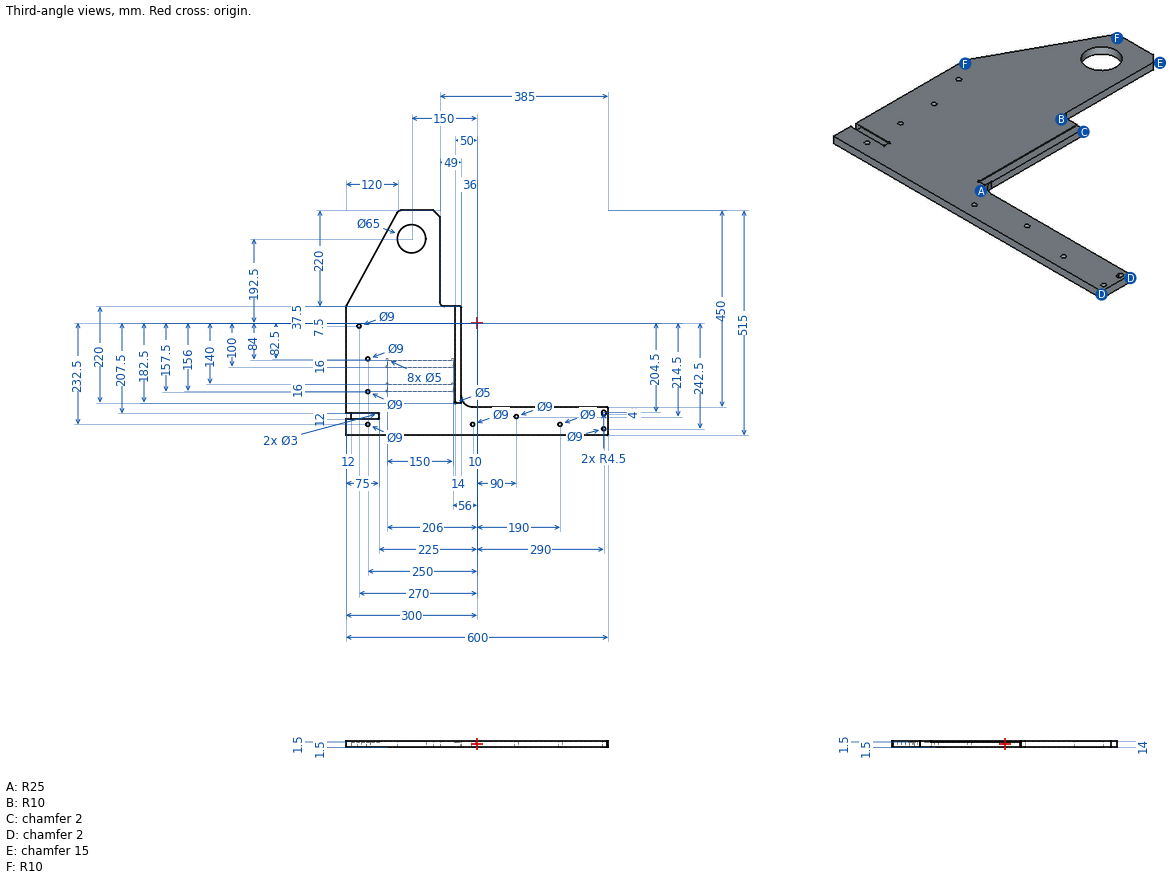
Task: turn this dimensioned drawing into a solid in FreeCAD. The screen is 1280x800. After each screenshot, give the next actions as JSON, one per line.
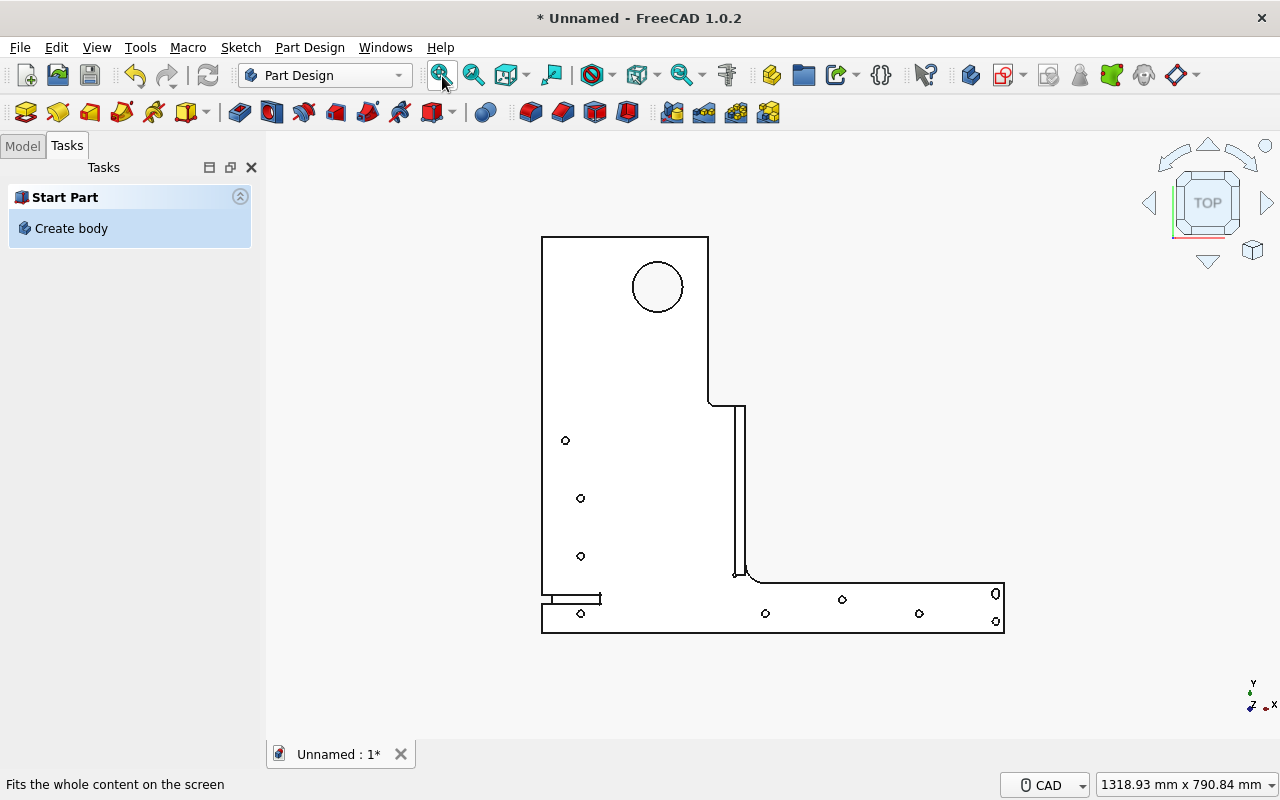
{"action": "key", "text": "0"}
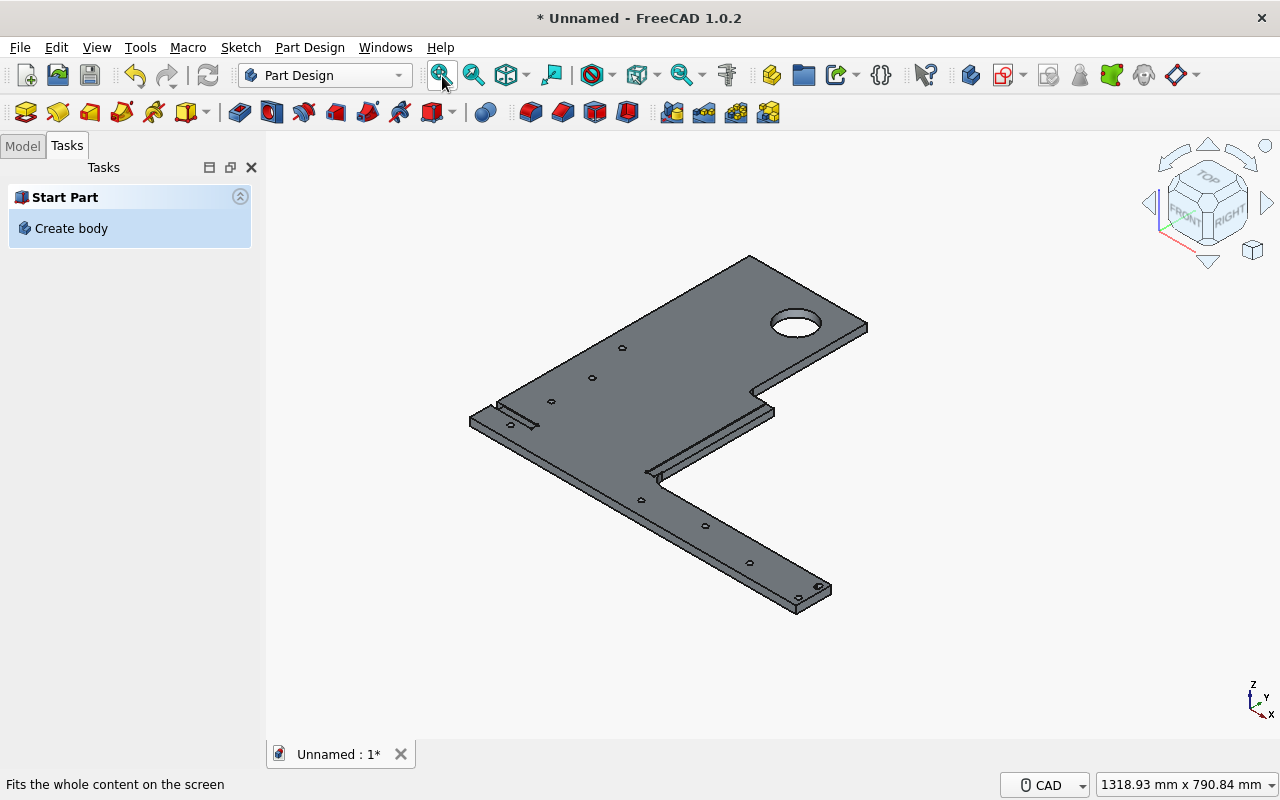
{"action": "scroll", "coordinate": [774, 411], "scroll_direction": "up", "scroll_amount": 8}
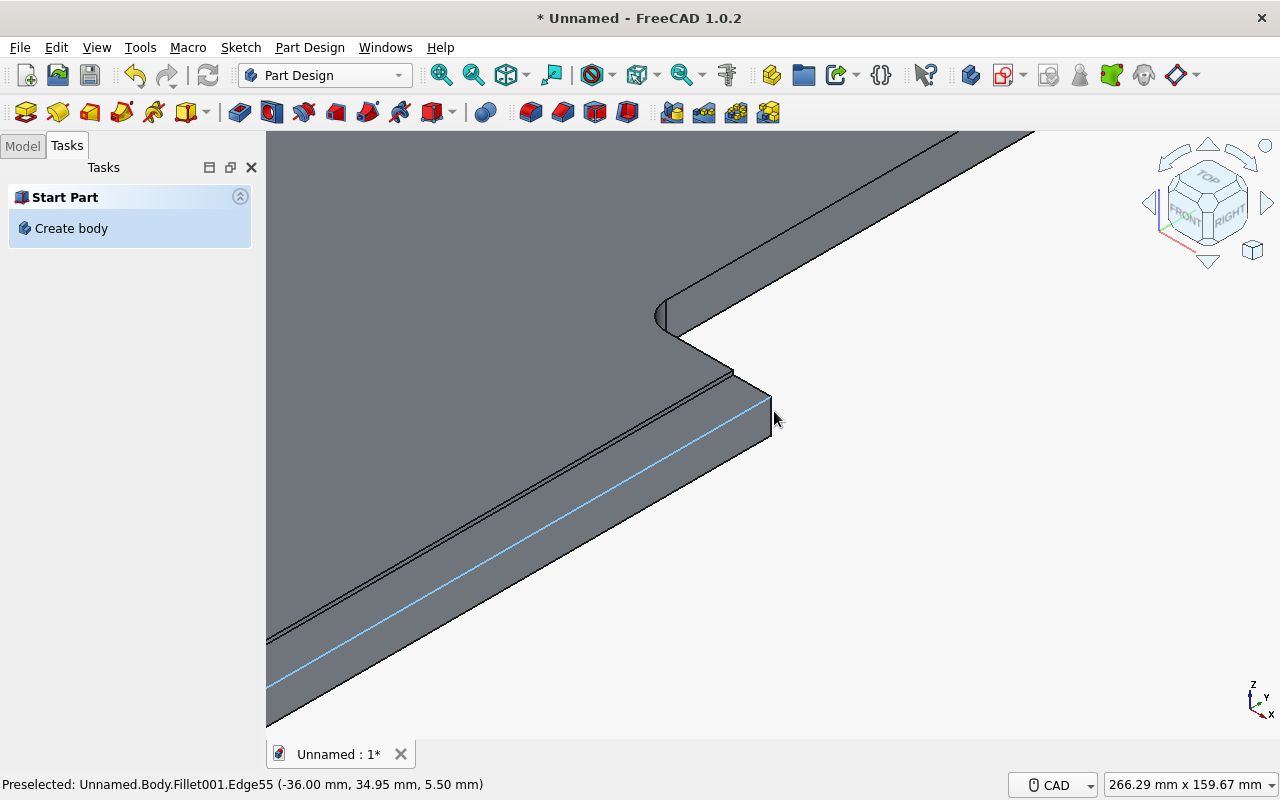
{"action": "left_click", "coordinate": [442, 76]}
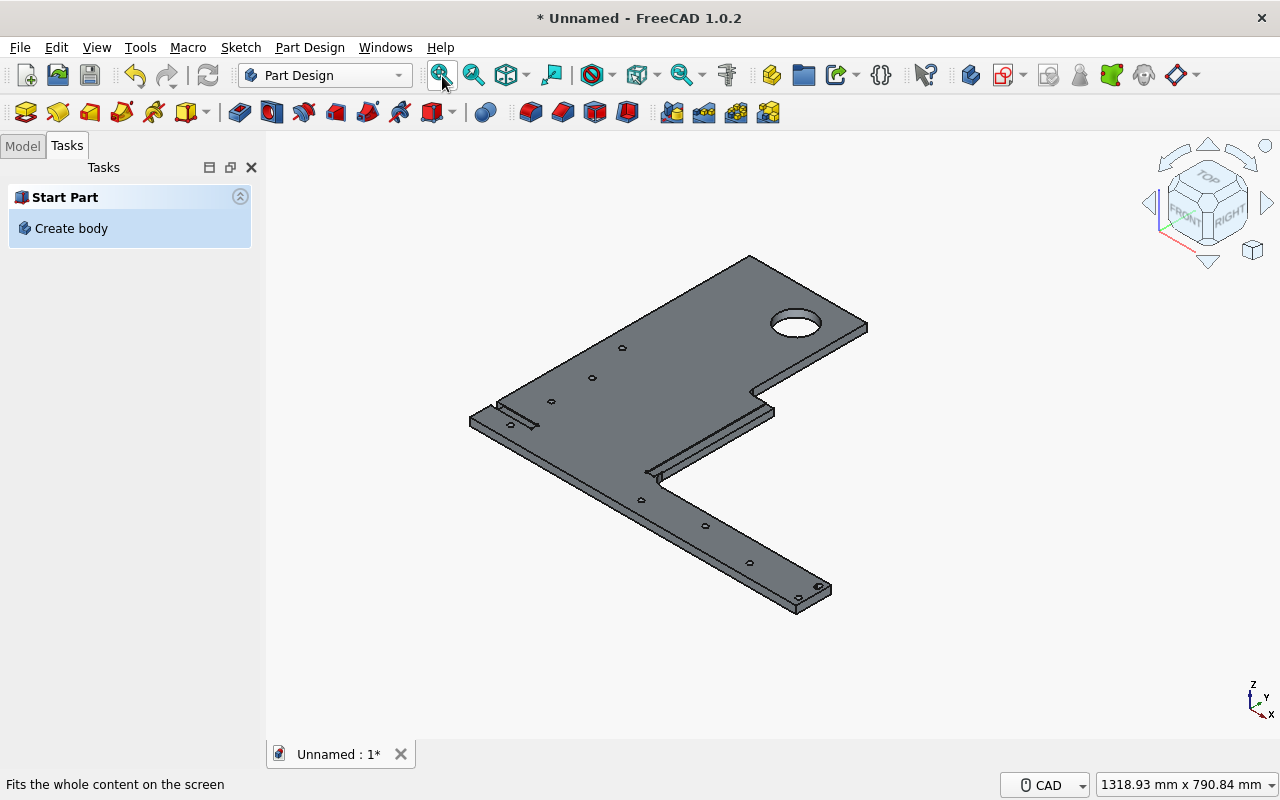
{"action": "key", "text": "1"}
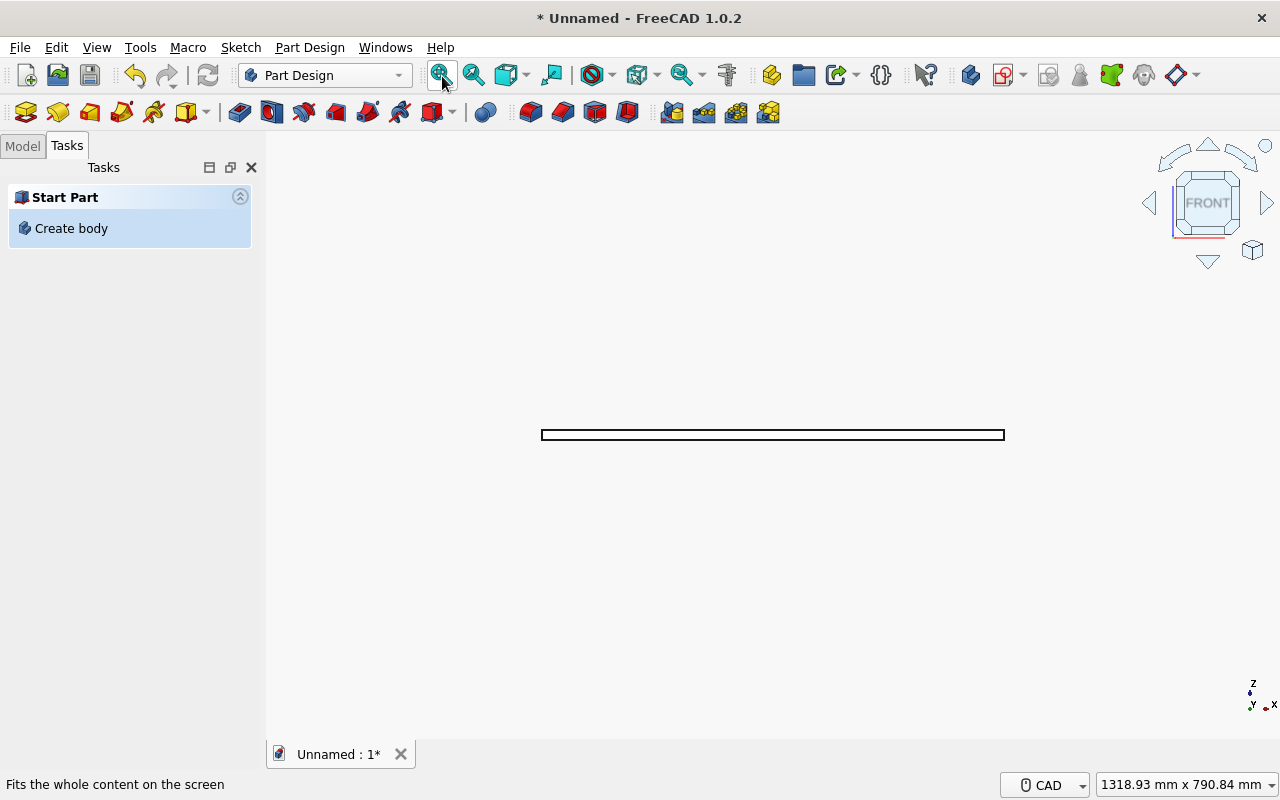
{"action": "scroll", "coordinate": [745, 435], "scroll_direction": "up", "scroll_amount": 8}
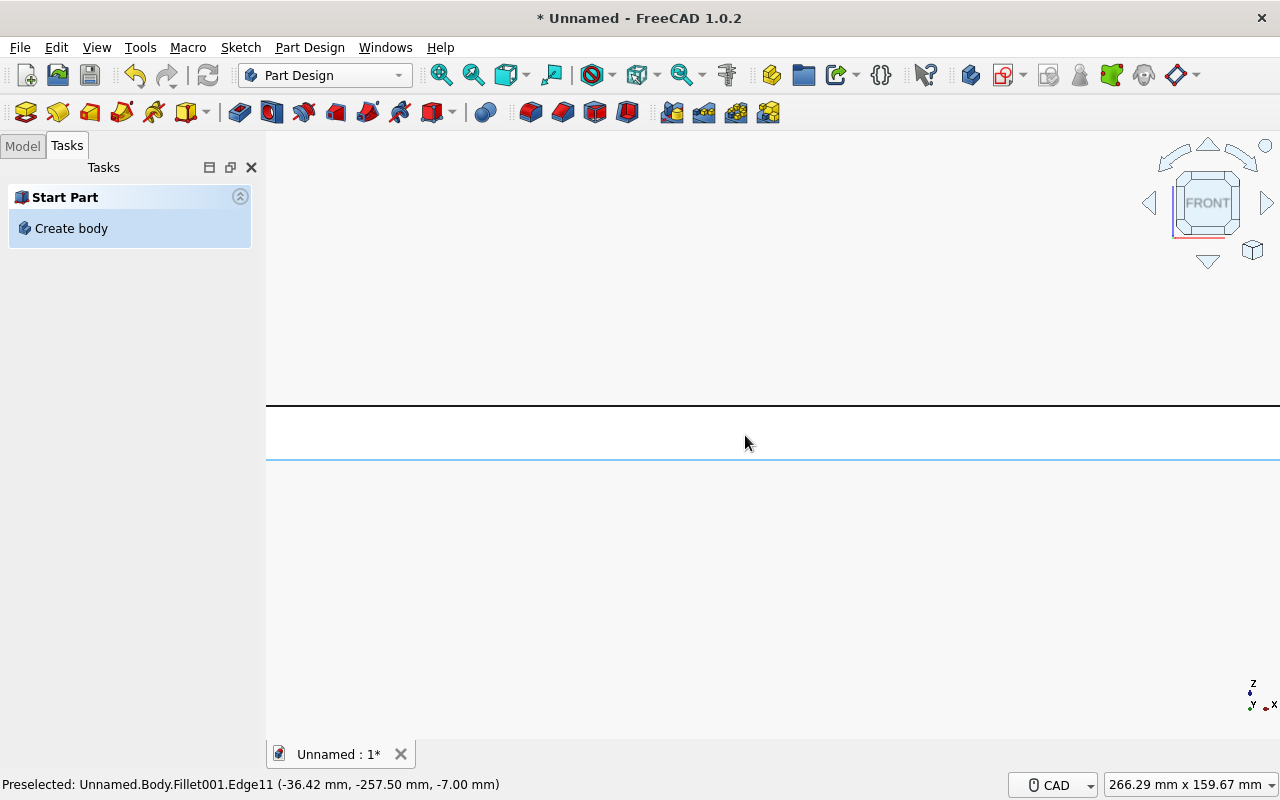
{"action": "left_click", "coordinate": [442, 76]}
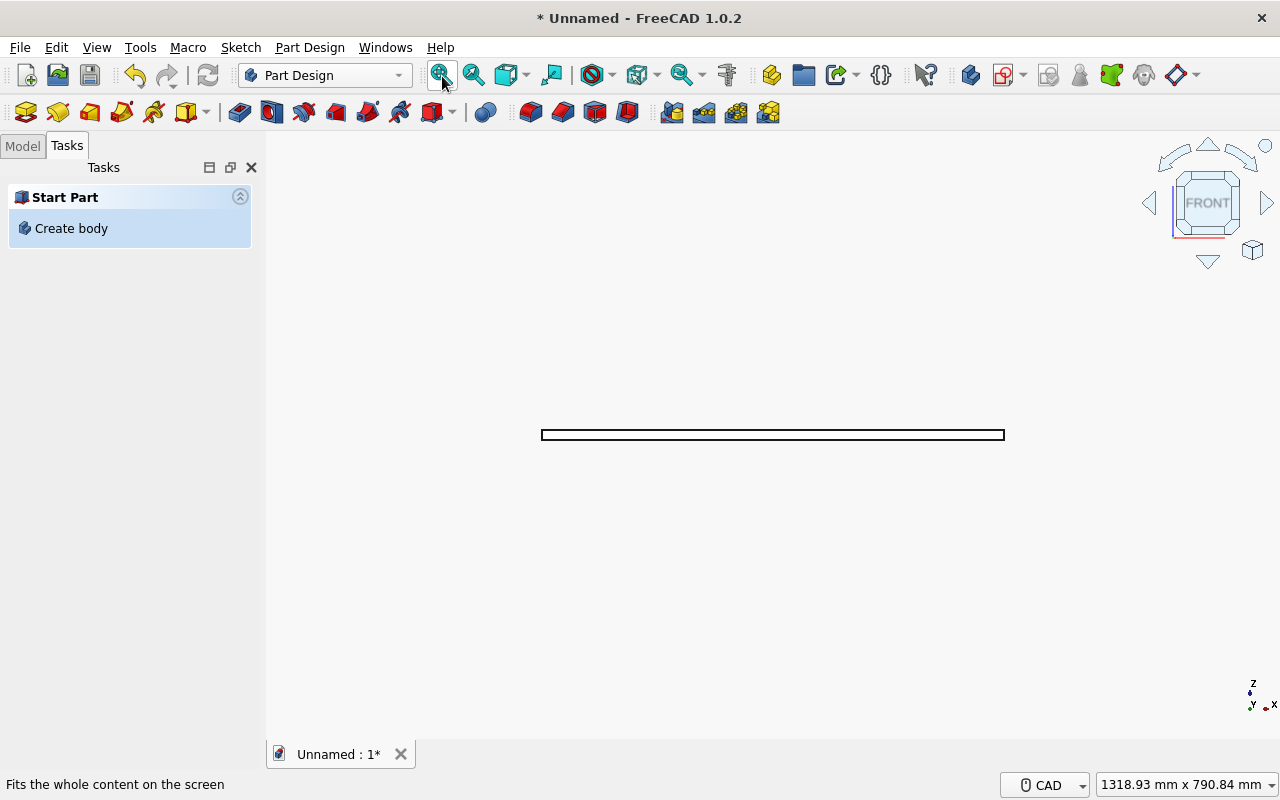
{"action": "key", "text": "3"}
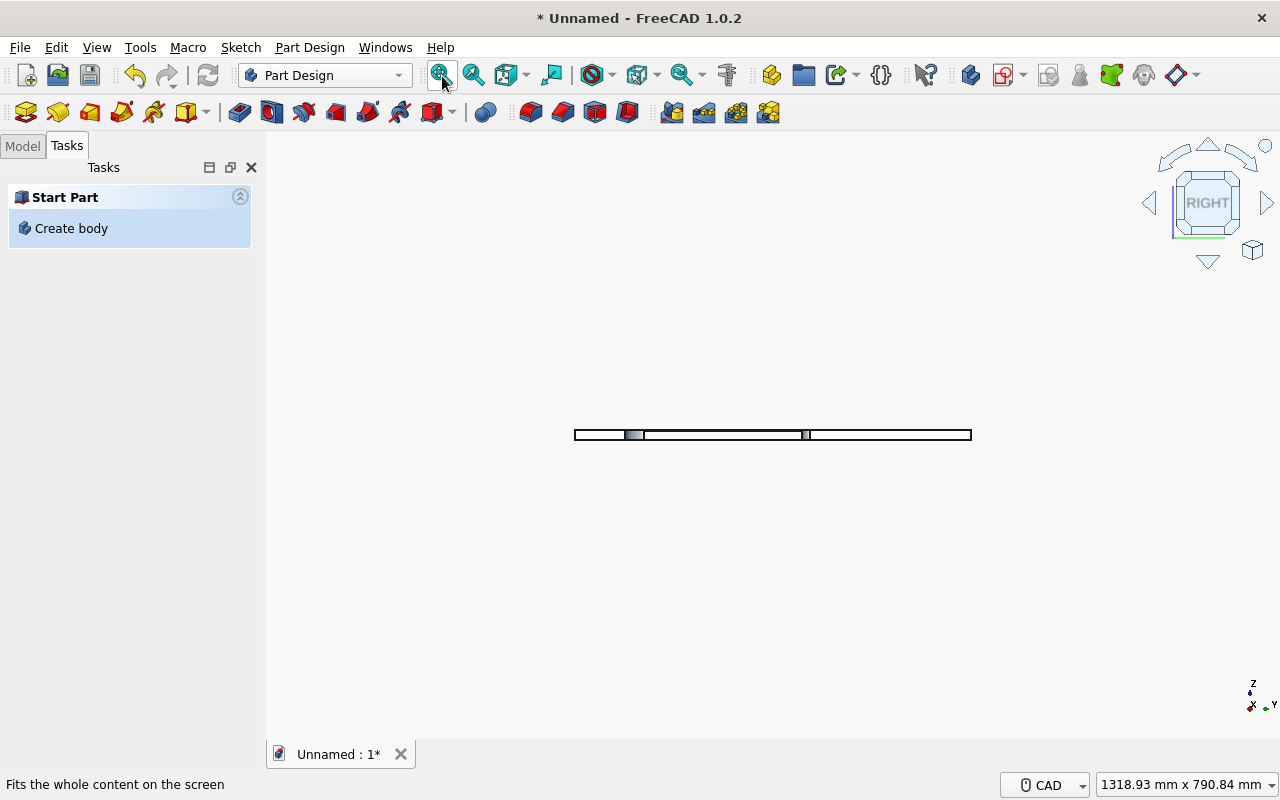
{"action": "left_click", "coordinate": [442, 76]}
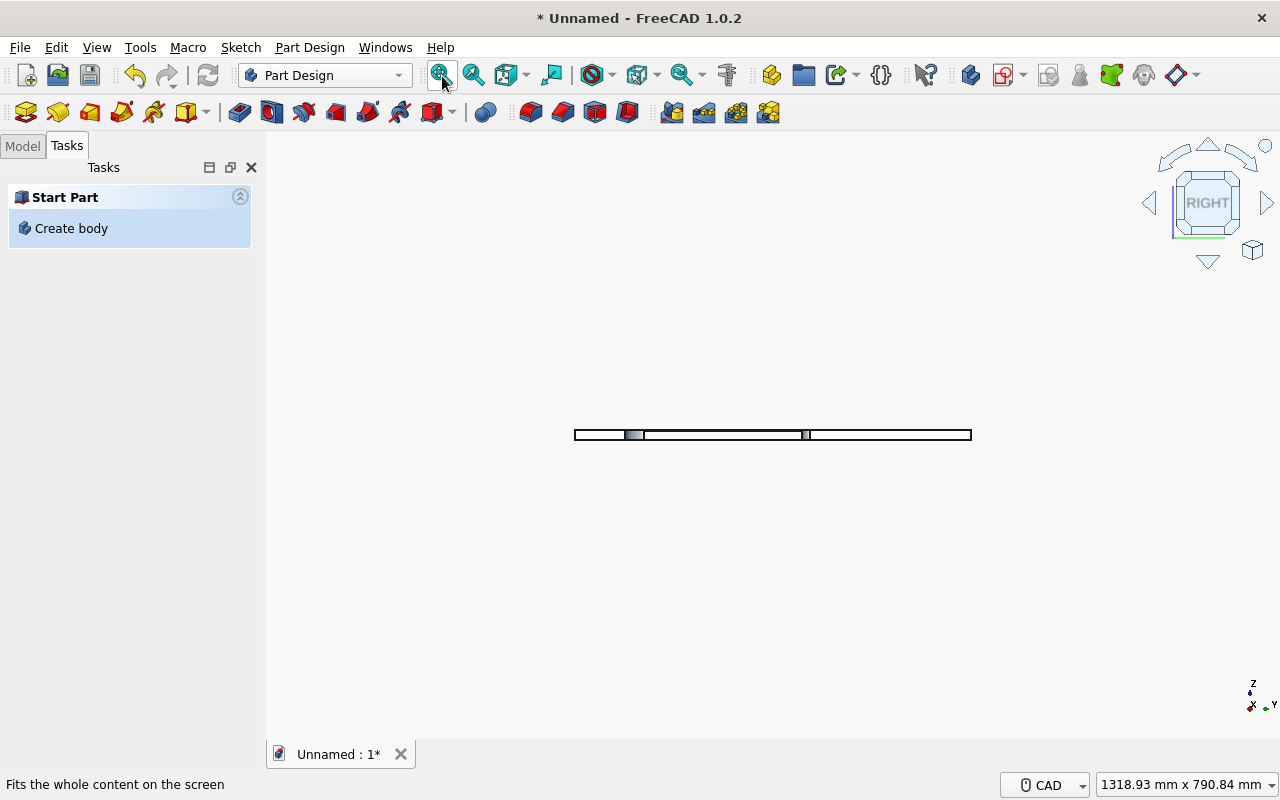
{"action": "scroll", "coordinate": [802, 435], "scroll_direction": "up", "scroll_amount": 8}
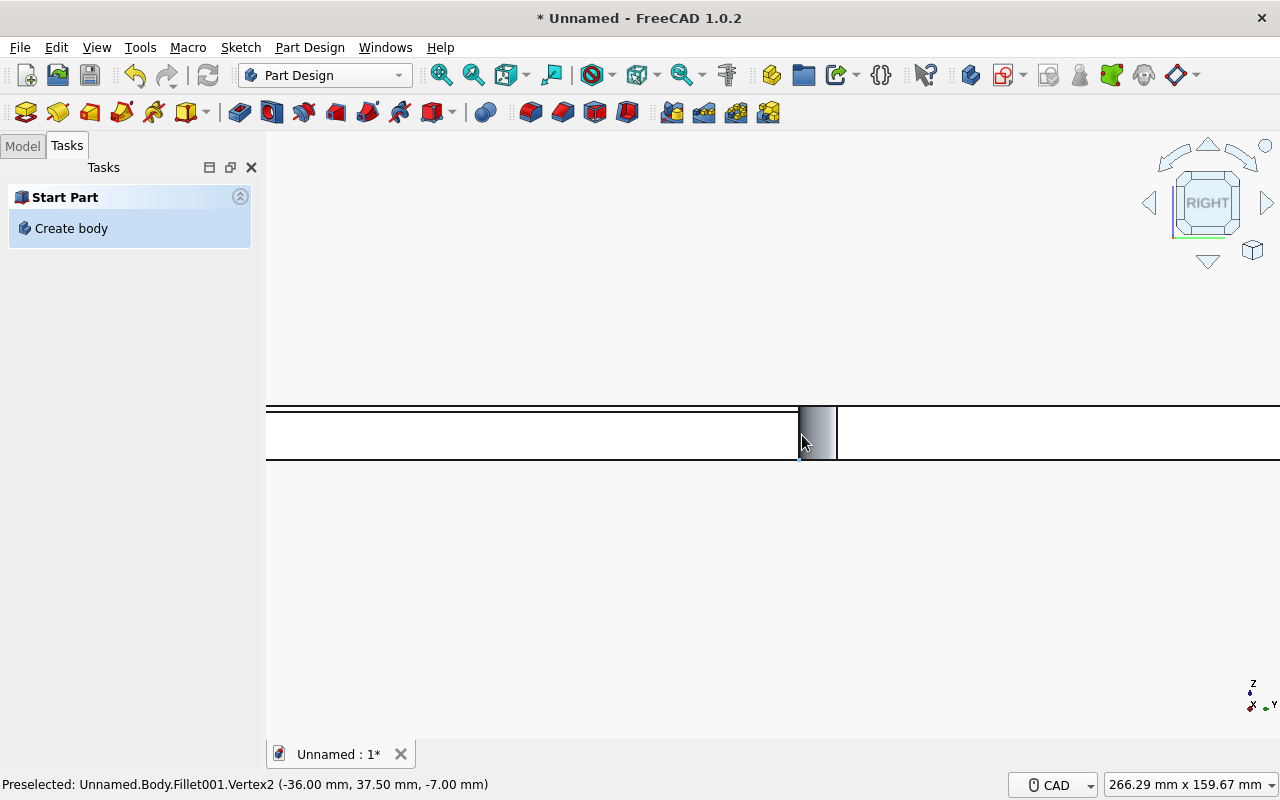
{"action": "left_click", "coordinate": [799, 435]}